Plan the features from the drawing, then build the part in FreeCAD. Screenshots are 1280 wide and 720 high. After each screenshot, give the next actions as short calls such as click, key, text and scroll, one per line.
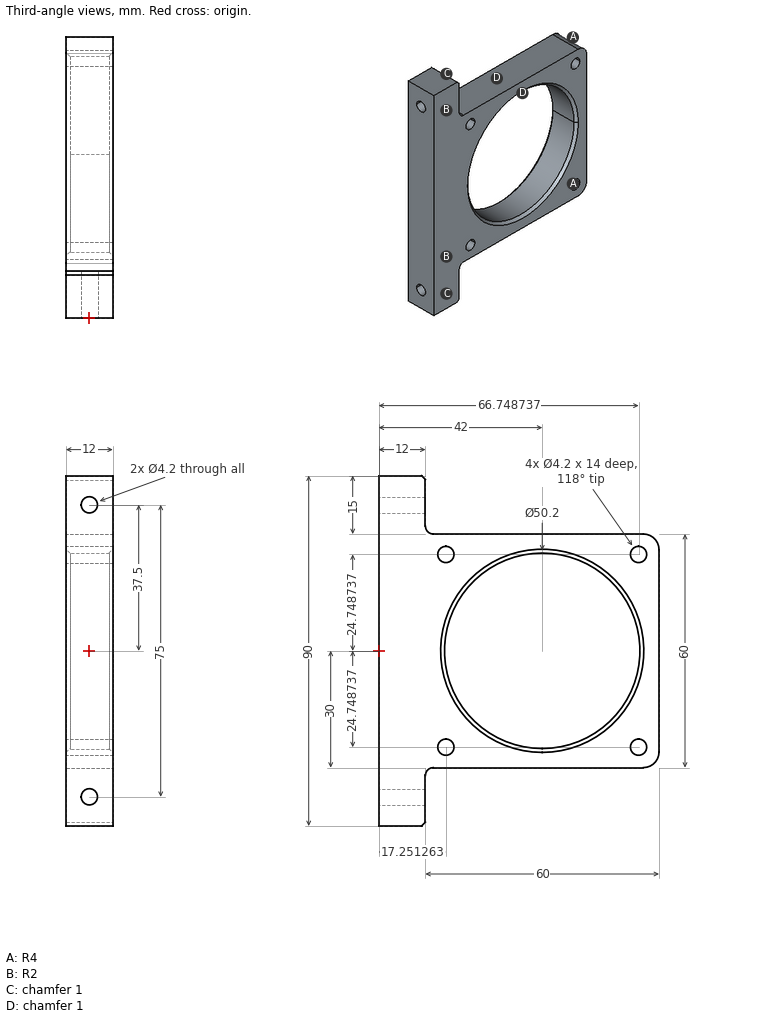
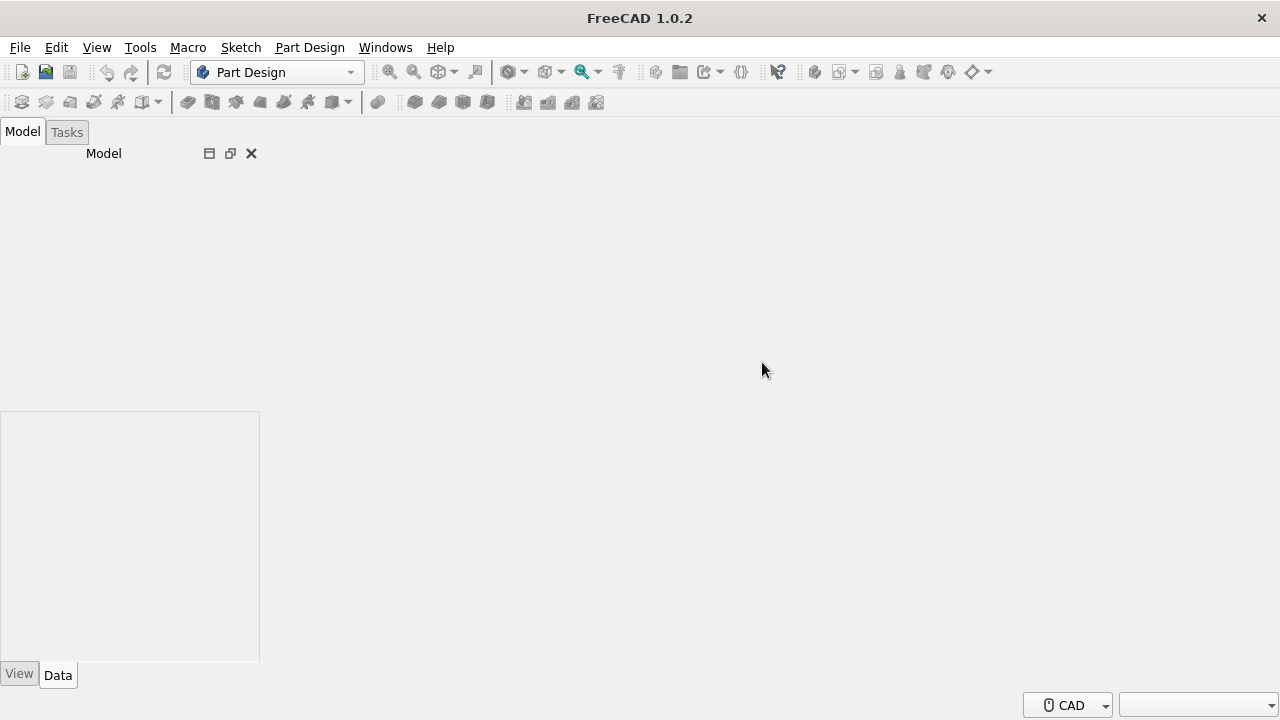
click(22, 72)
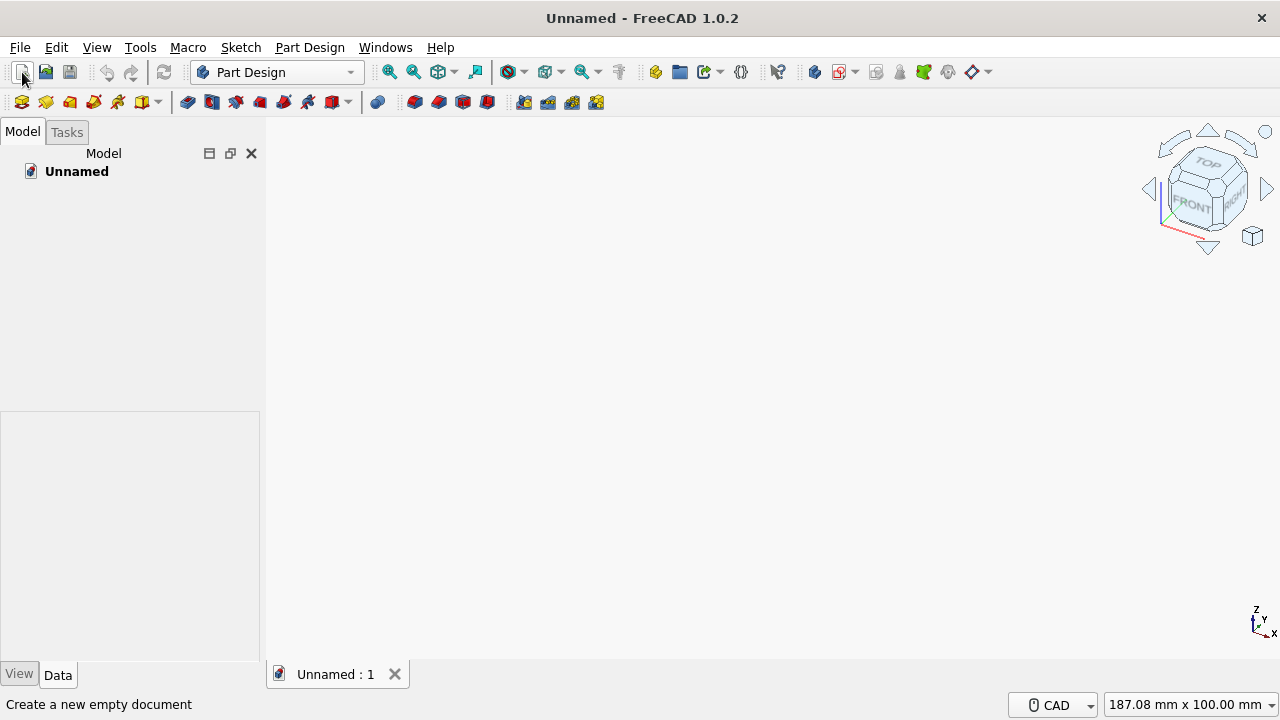
click(840, 72)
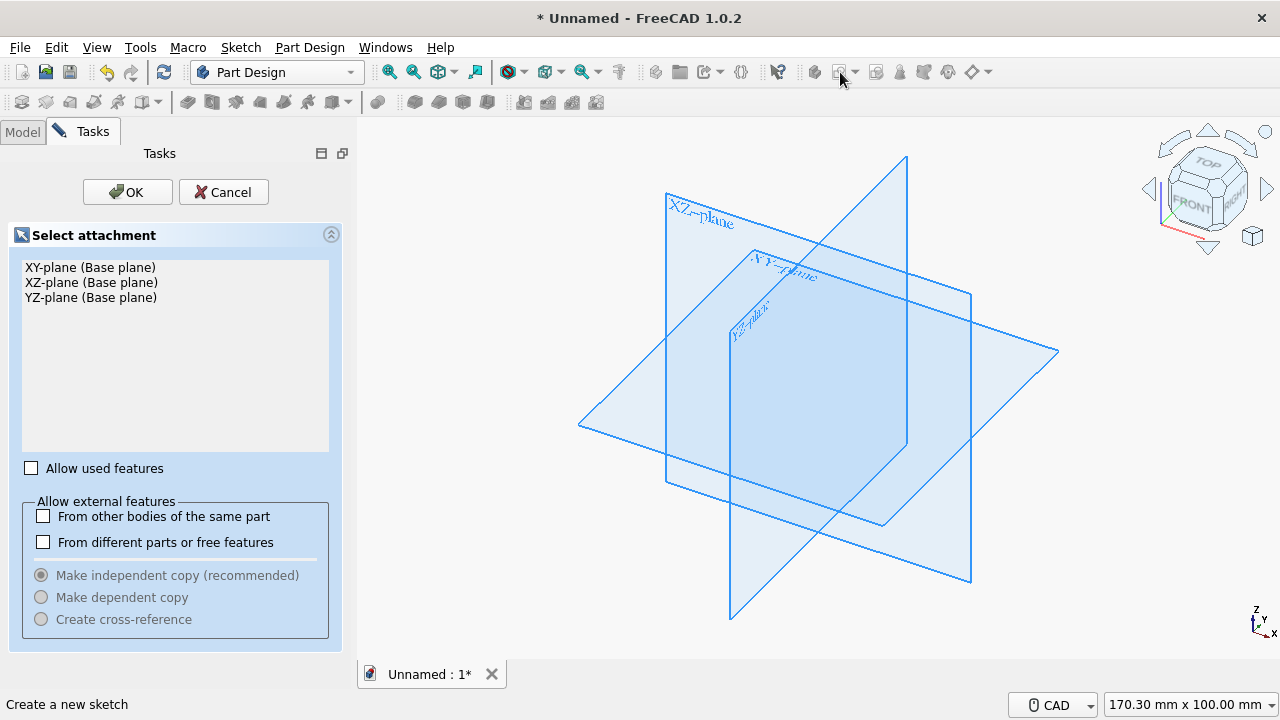
click(82, 298)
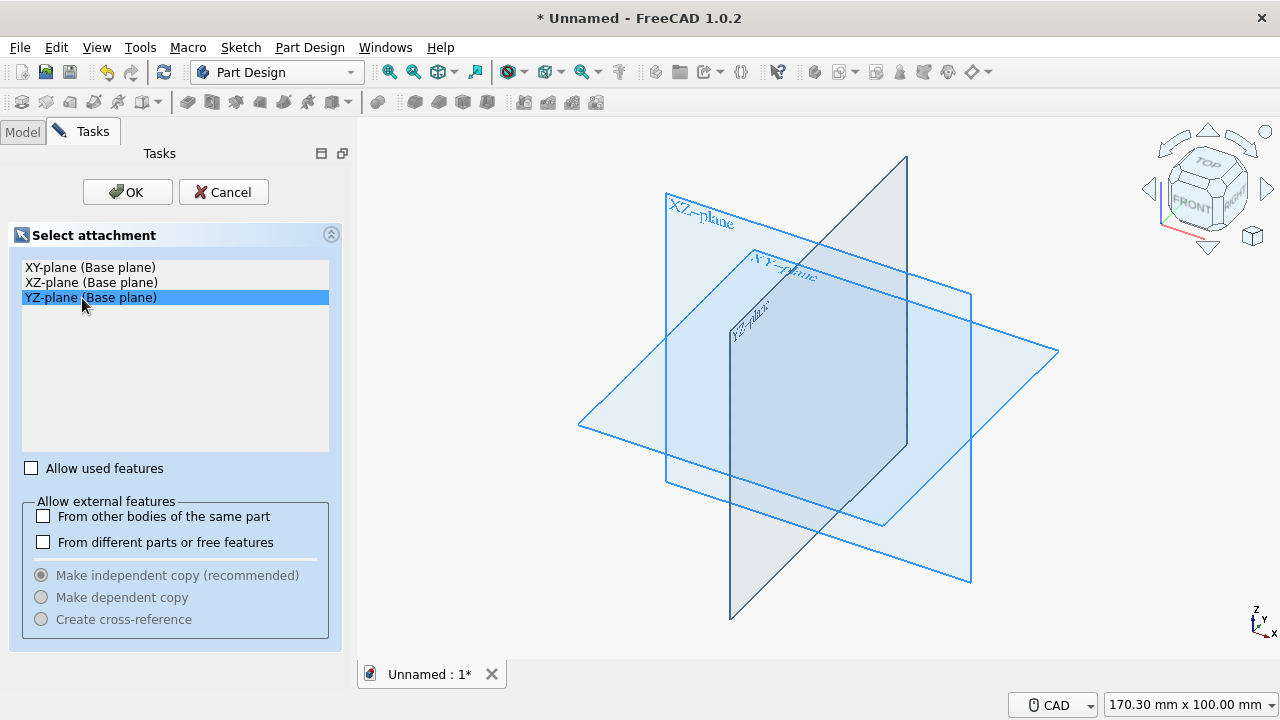
click(128, 192)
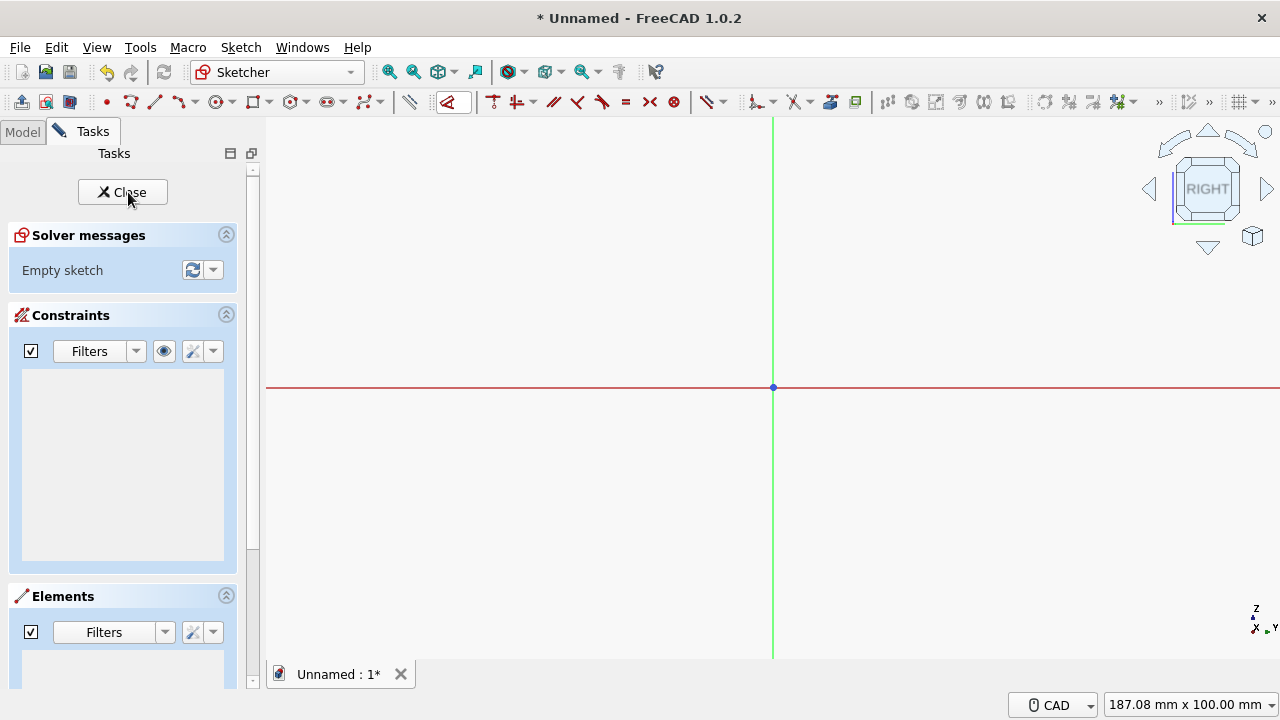
scroll(294, 388, down, 2)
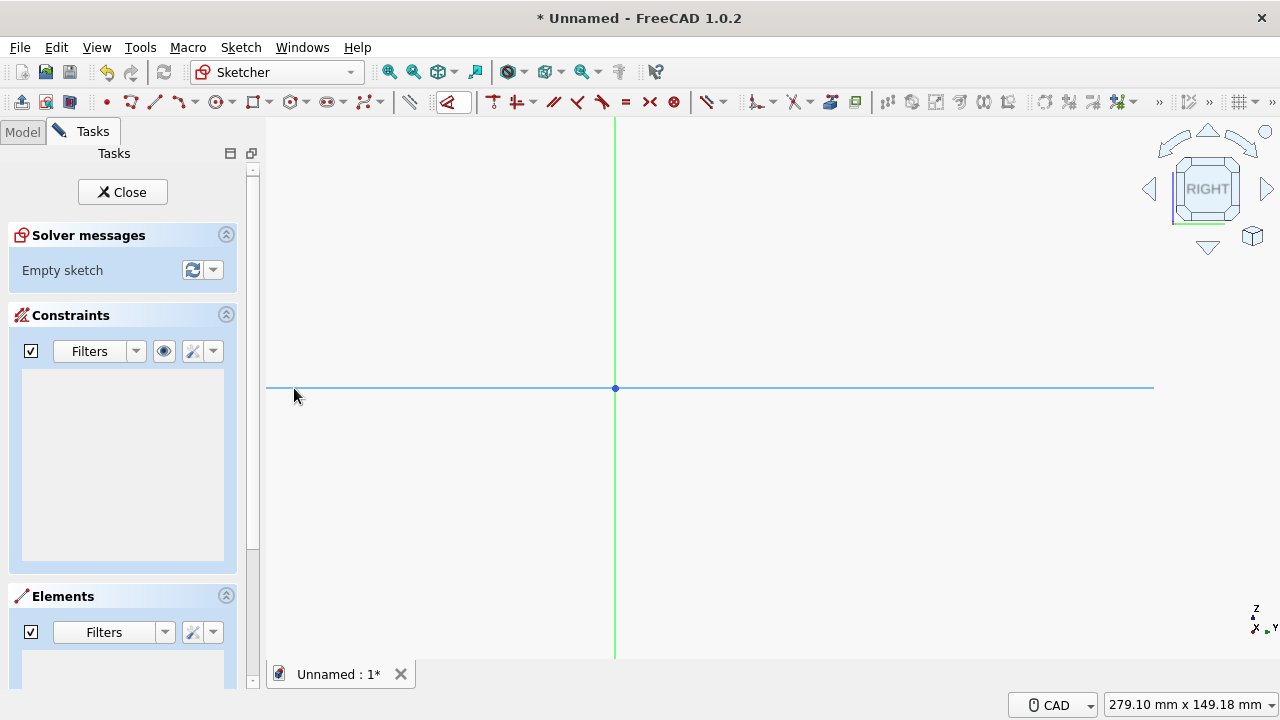
click(132, 102)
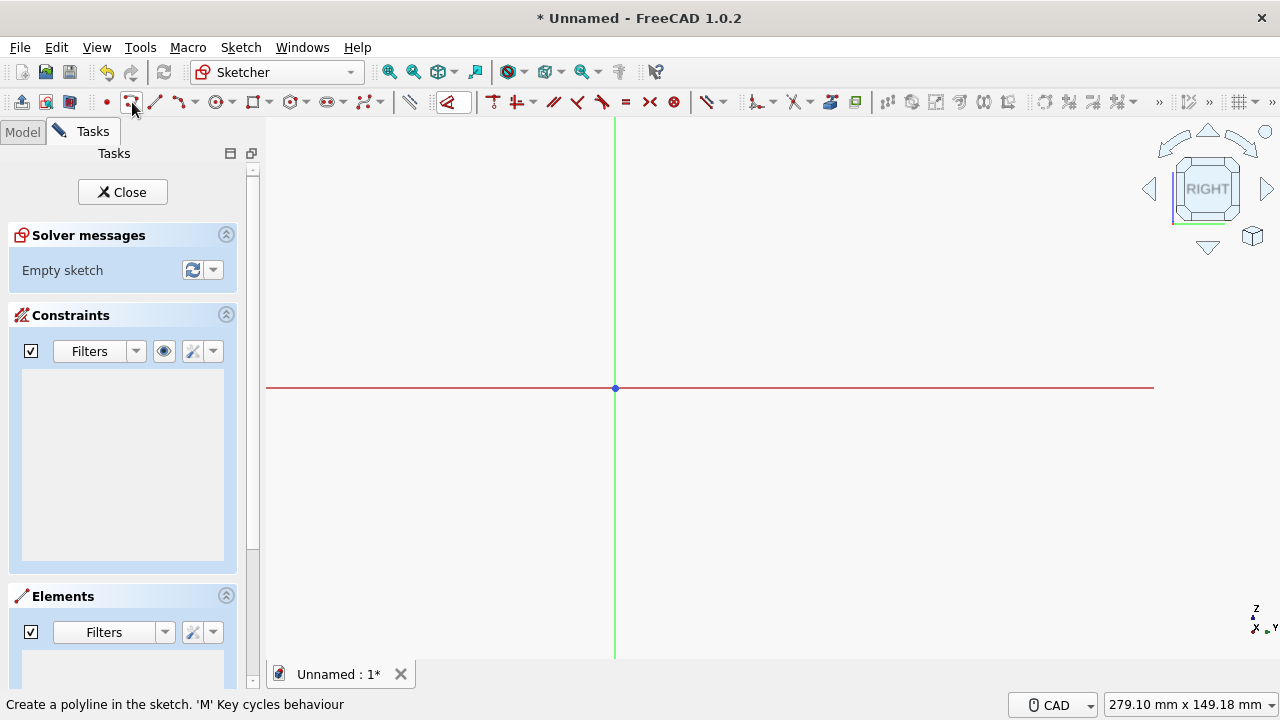
click(659, 497)
click(877, 497)
click(877, 279)
click(659, 279)
click(659, 225)
click(615, 225)
click(624, 552)
click(659, 552)
click(659, 498)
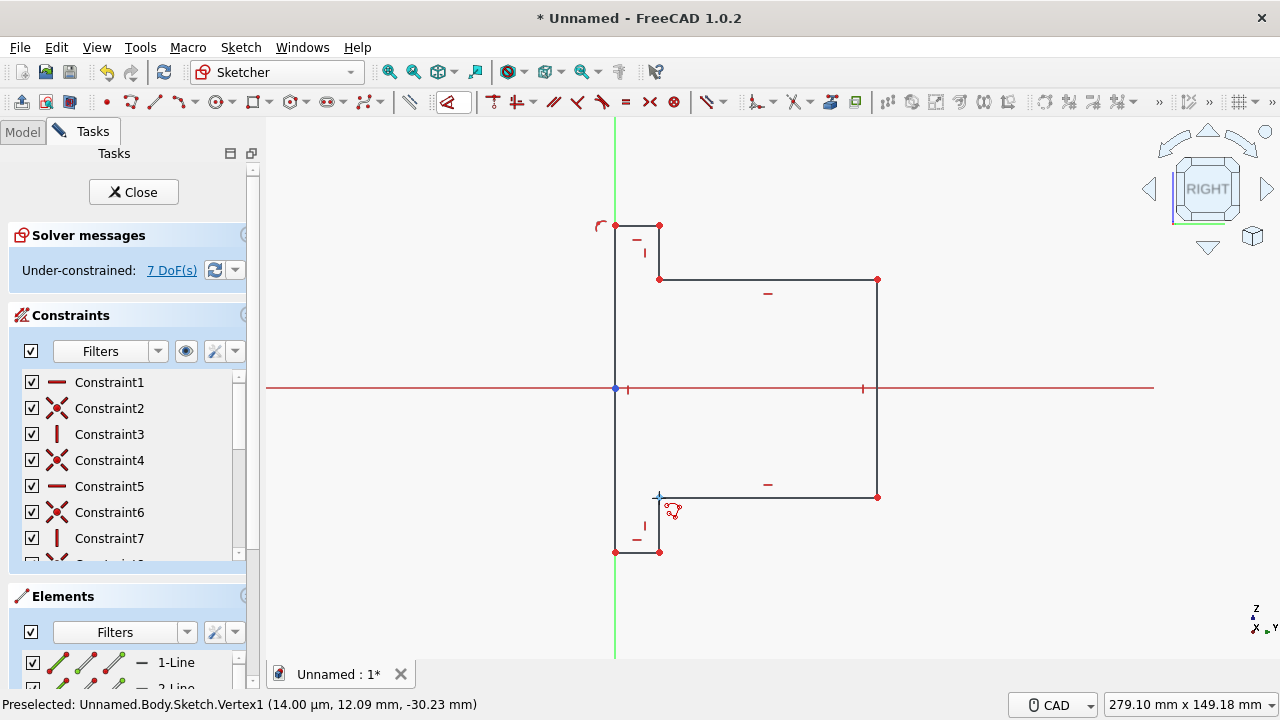
click(216, 102)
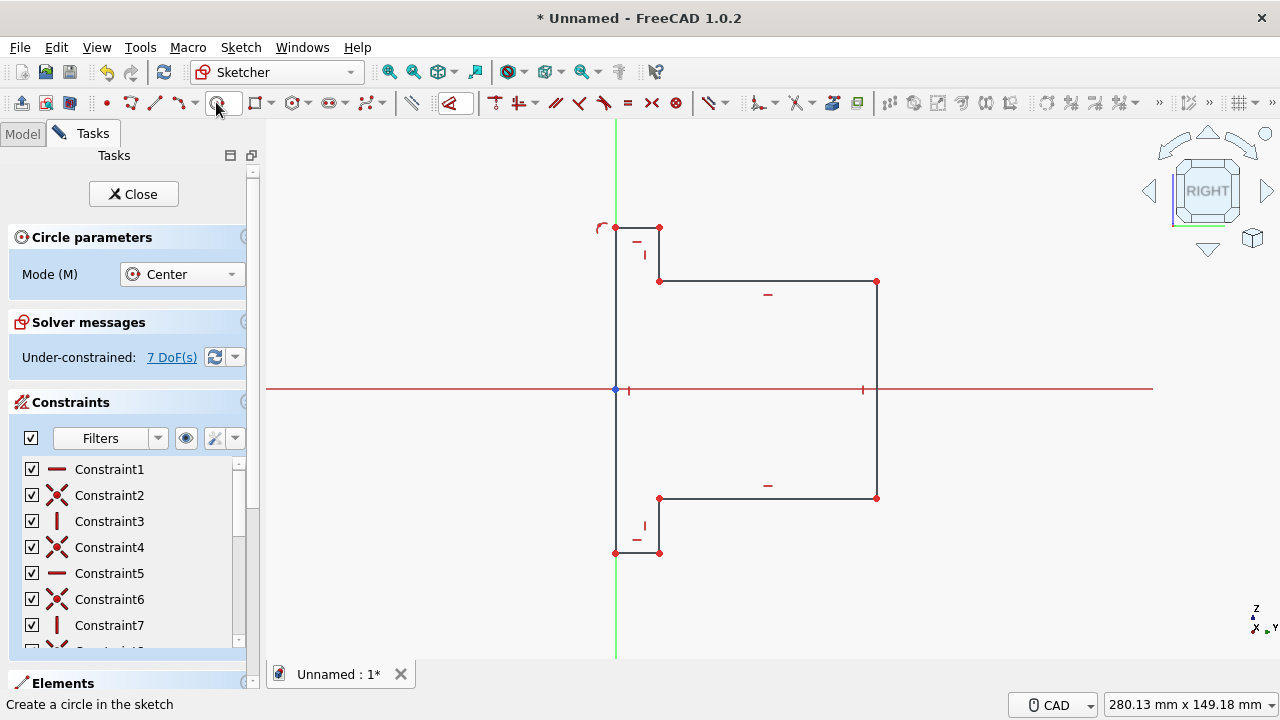
click(768, 389)
move(832, 325)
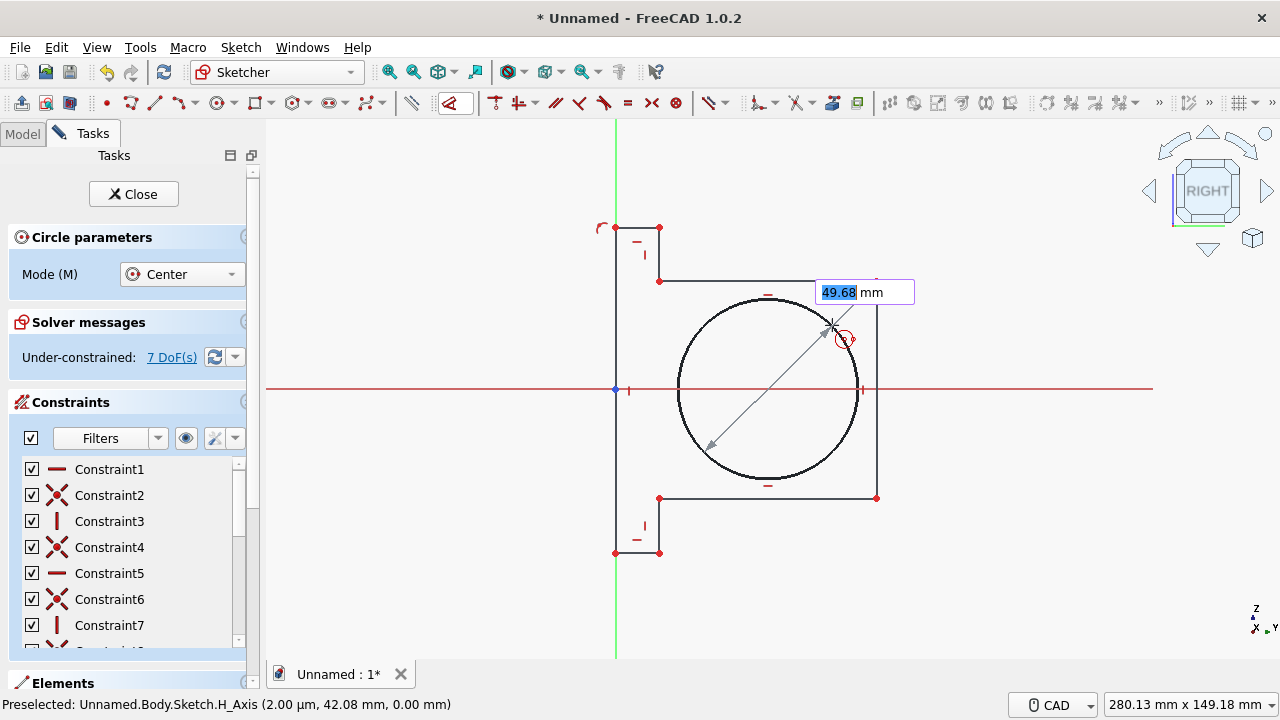
text(50.2)
key(Return)
key(Escape)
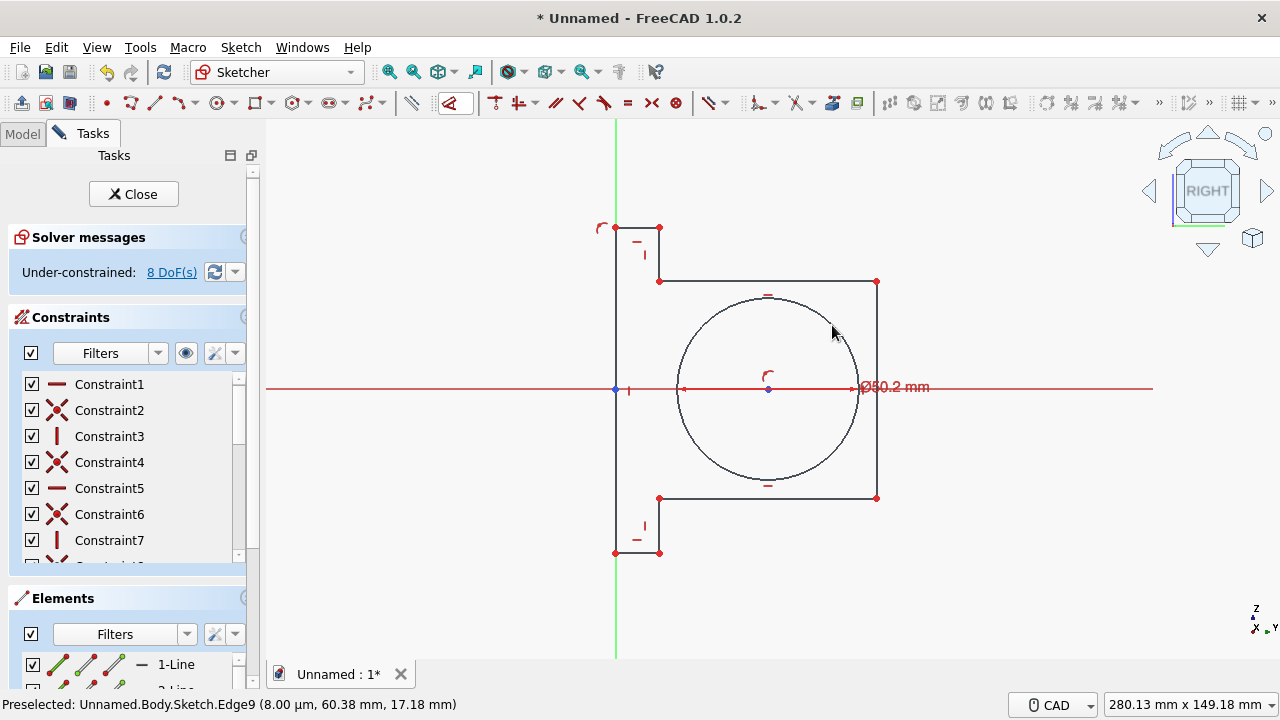
click(725, 499)